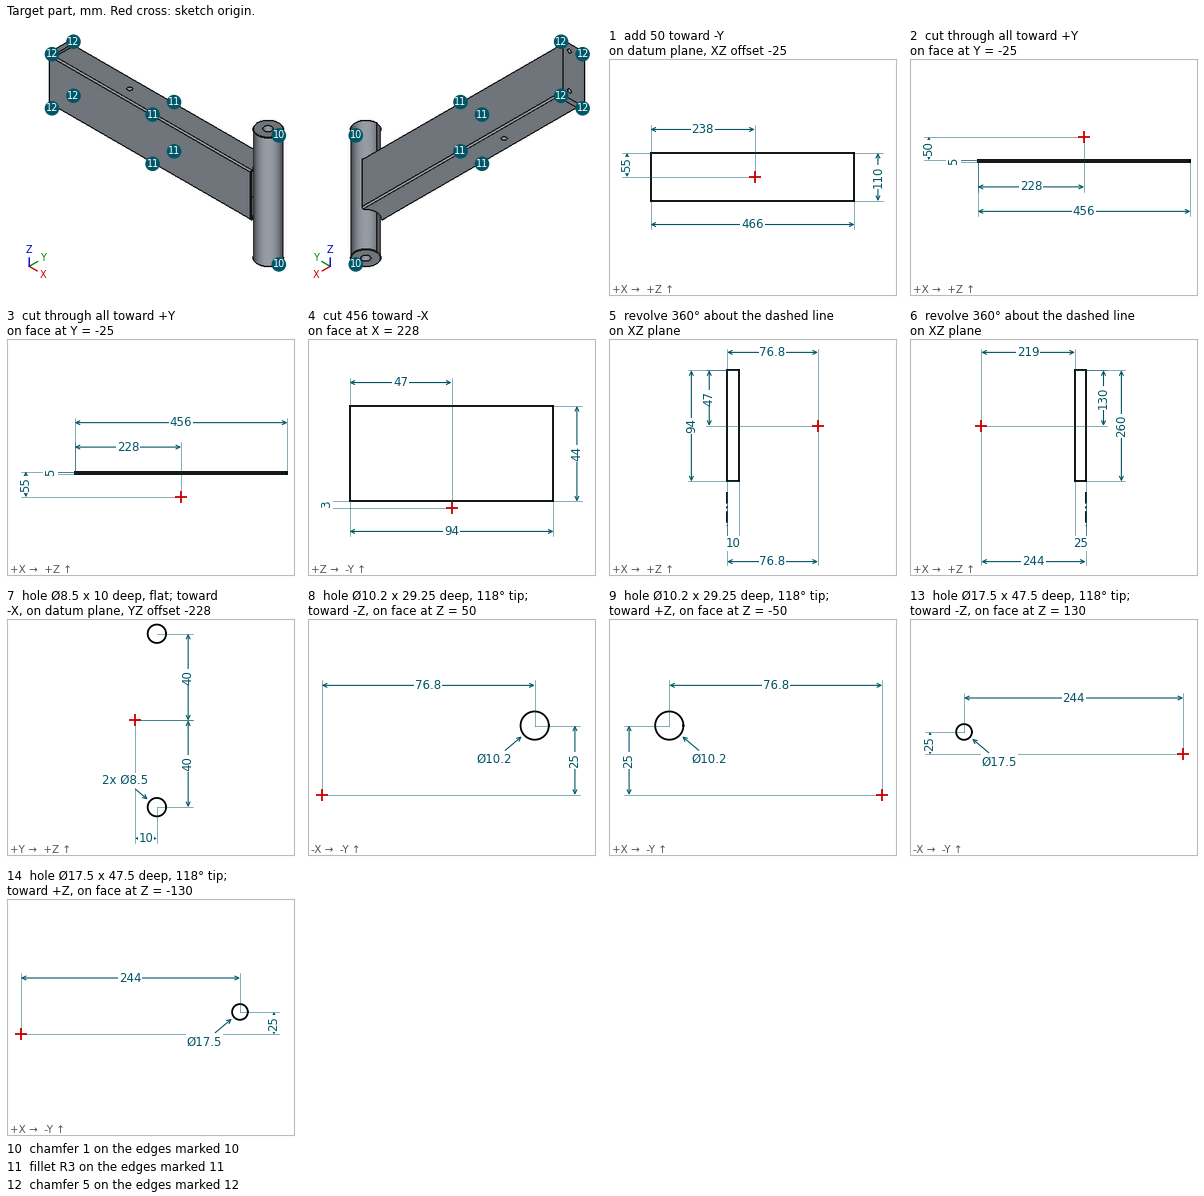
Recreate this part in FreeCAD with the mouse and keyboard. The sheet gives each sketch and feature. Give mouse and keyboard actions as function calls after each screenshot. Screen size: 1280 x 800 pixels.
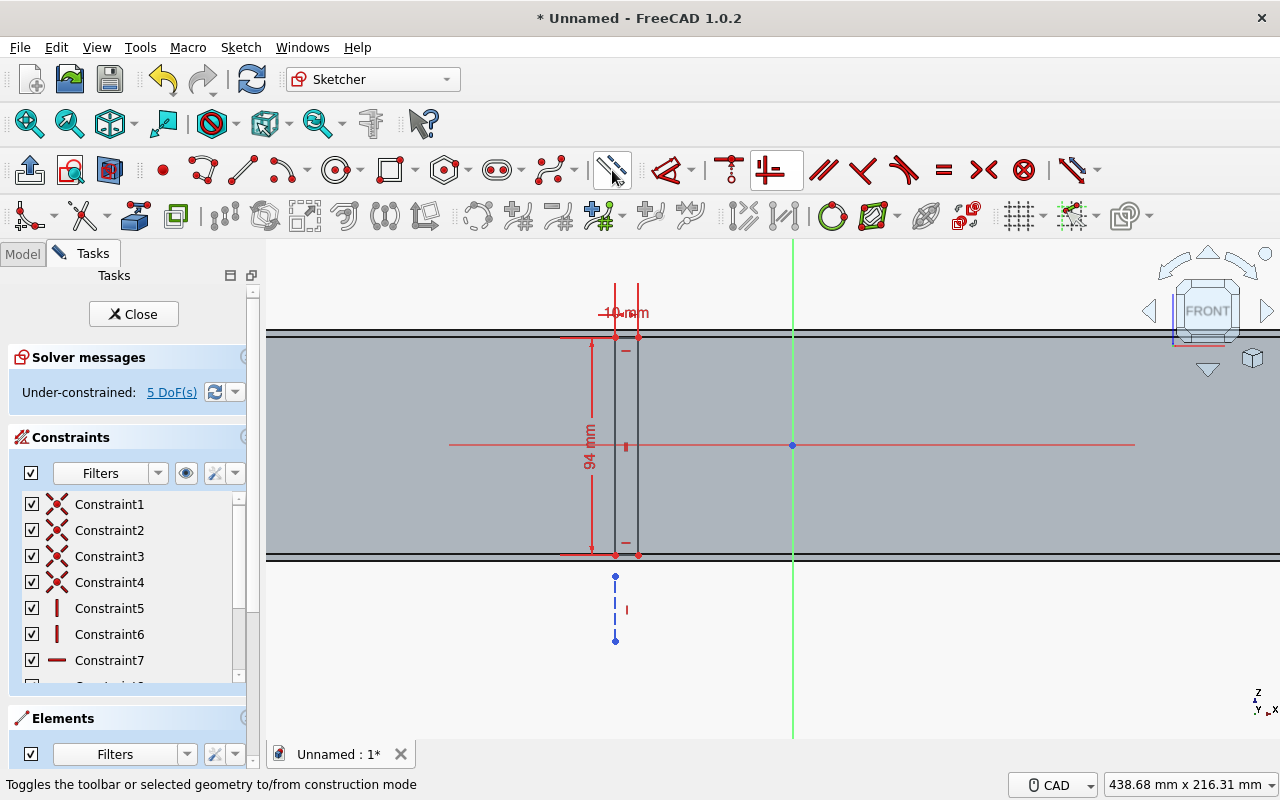
click(666, 170)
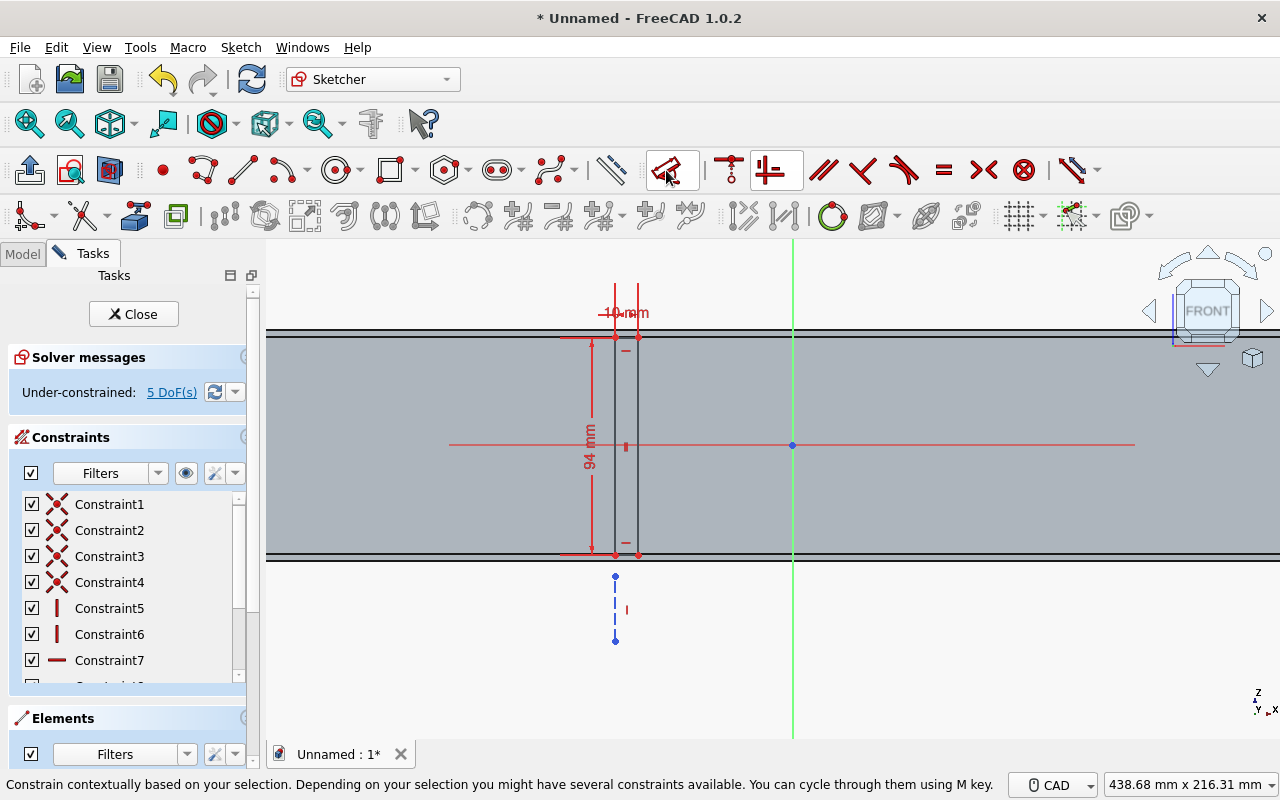
click(615, 338)
click(581, 392)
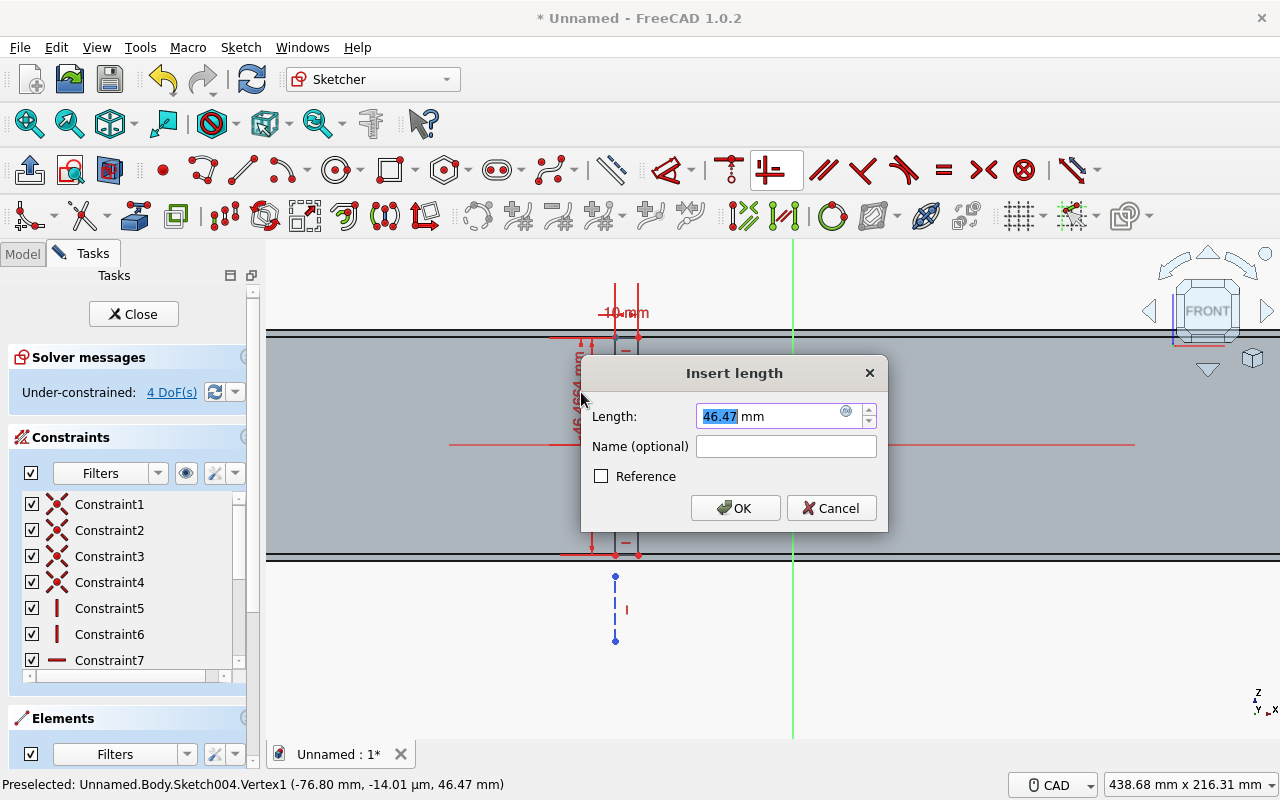
text(47)
key(Return)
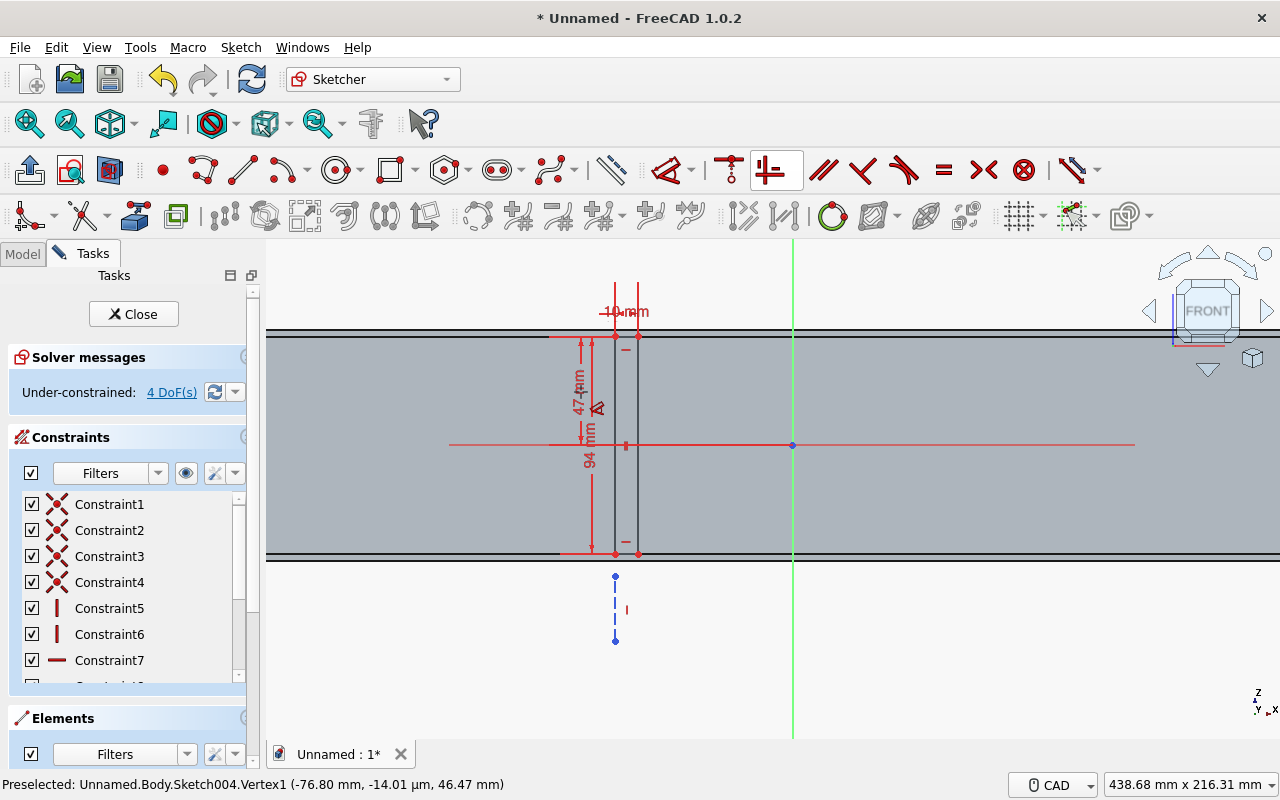
click(615, 337)
click(704, 303)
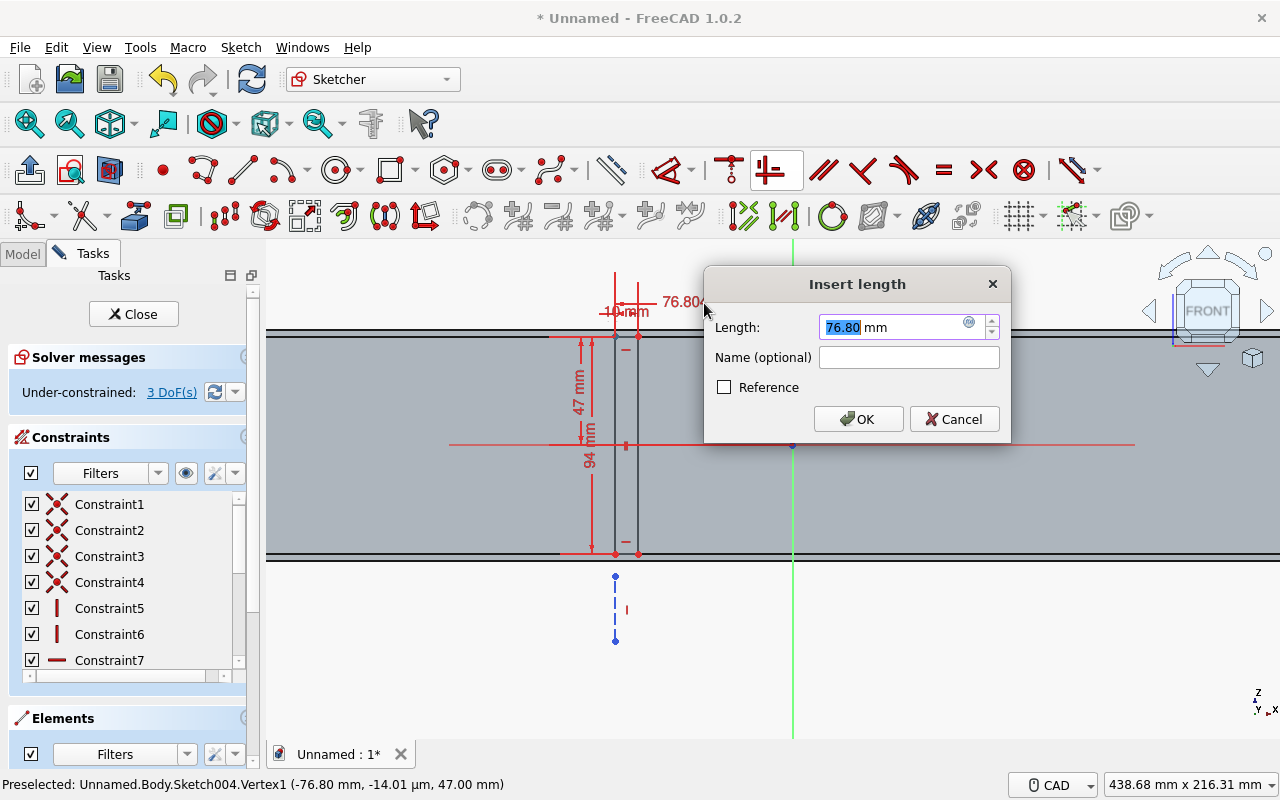
text(76.8)
key(Return)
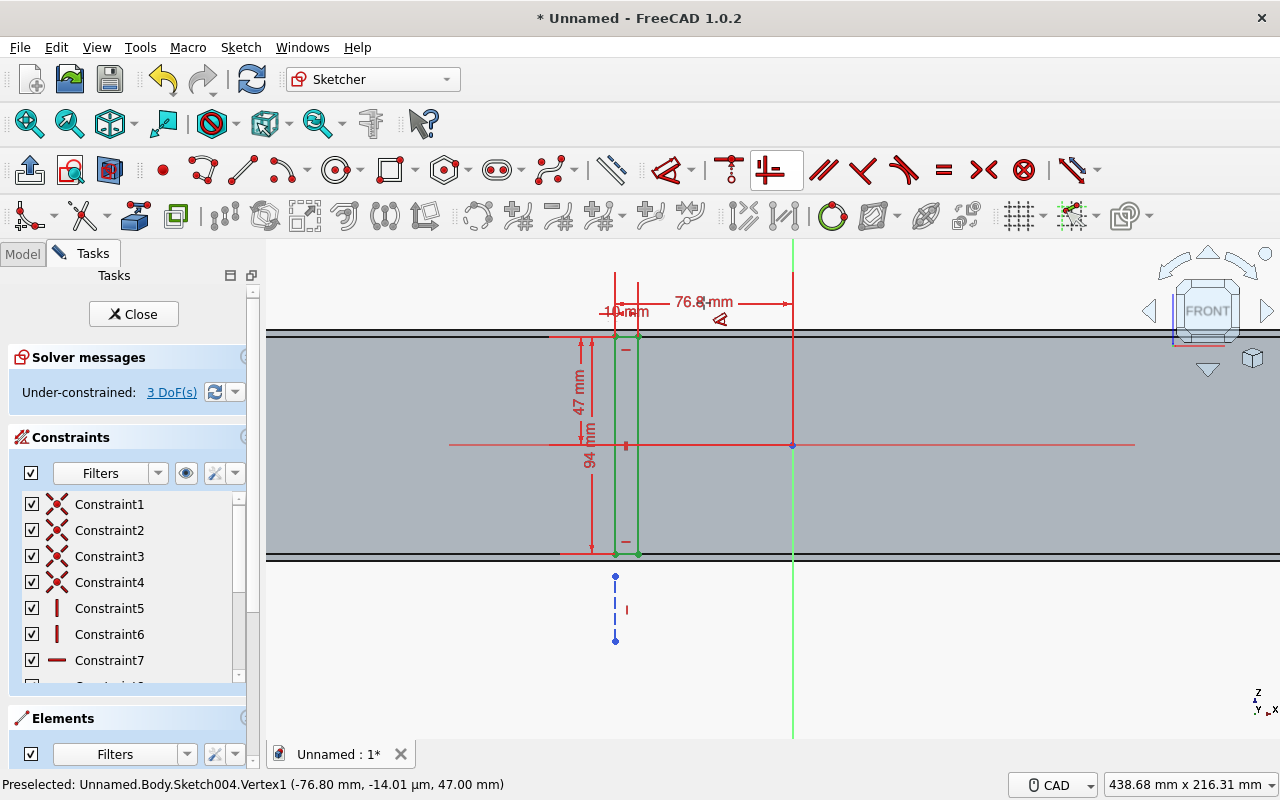
click(615, 577)
click(704, 611)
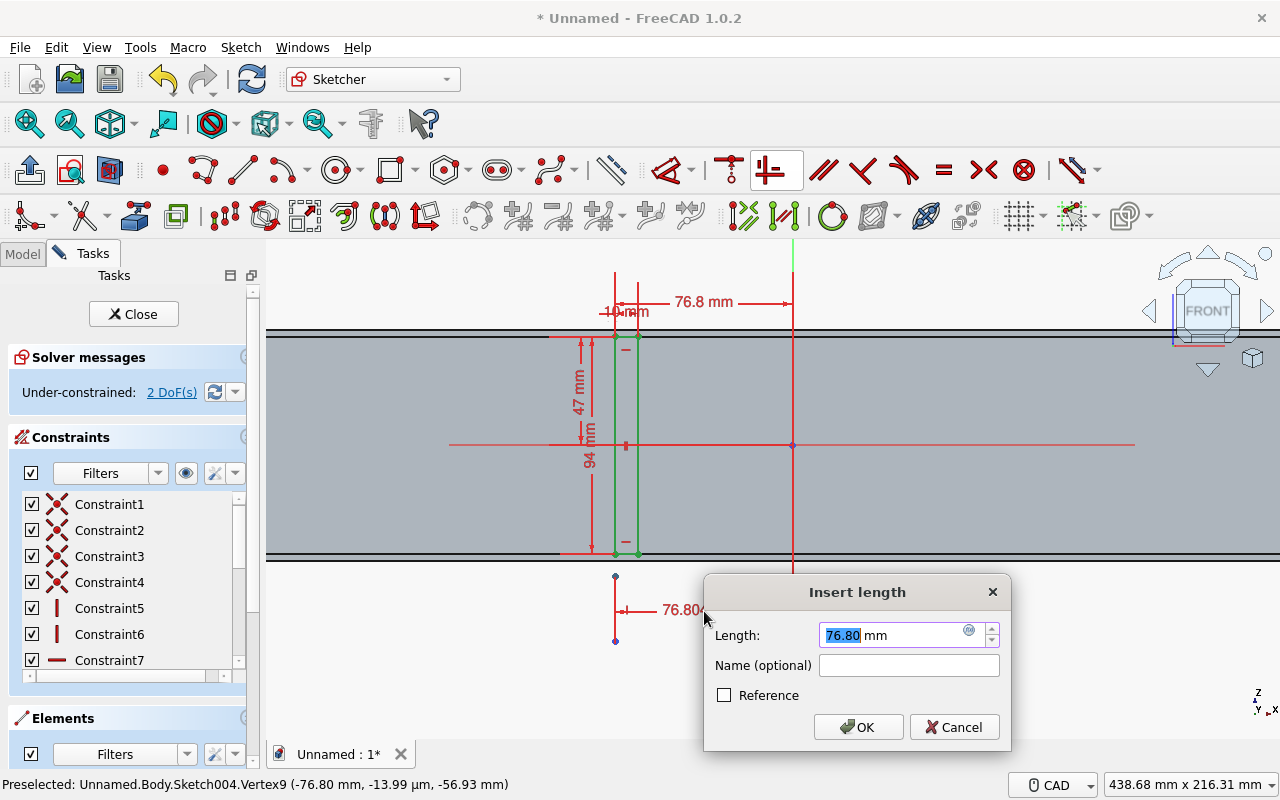
text(76.8)
key(Return)
key(Escape)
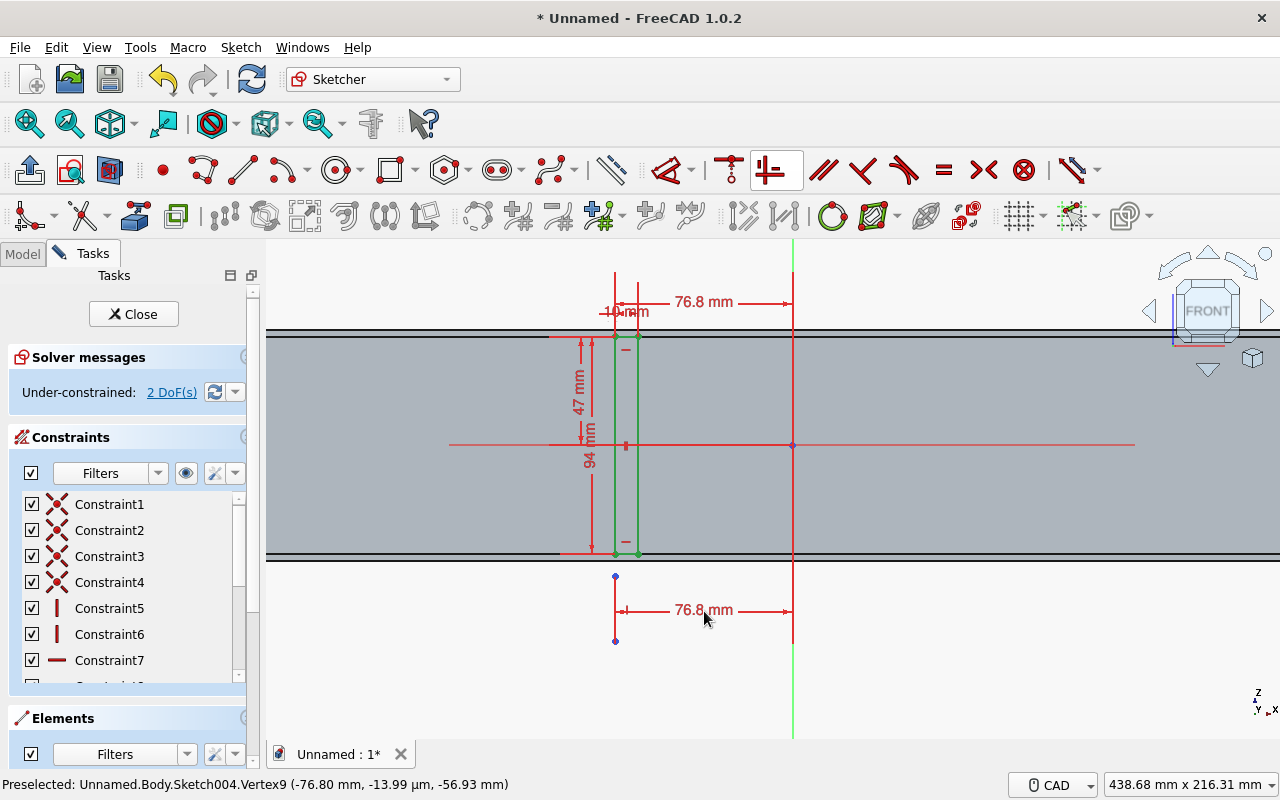
click(134, 314)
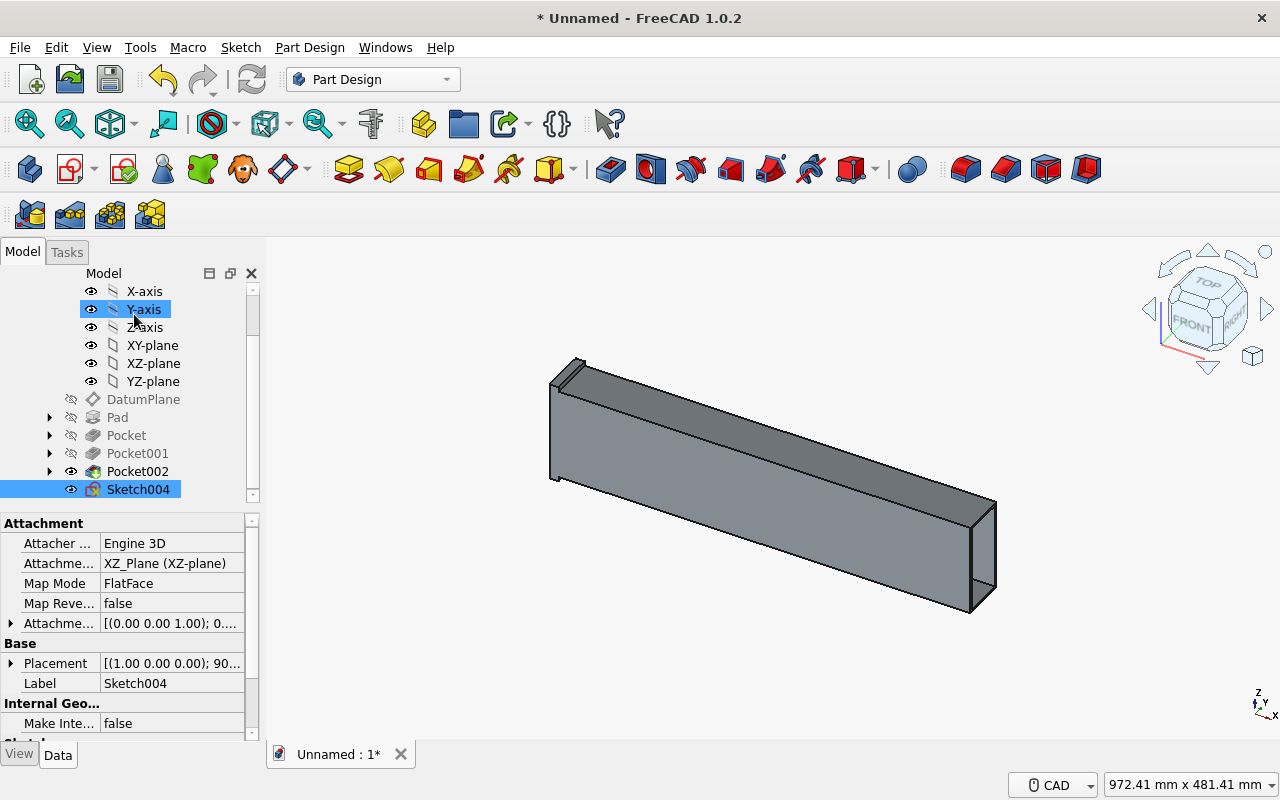
click(390, 170)